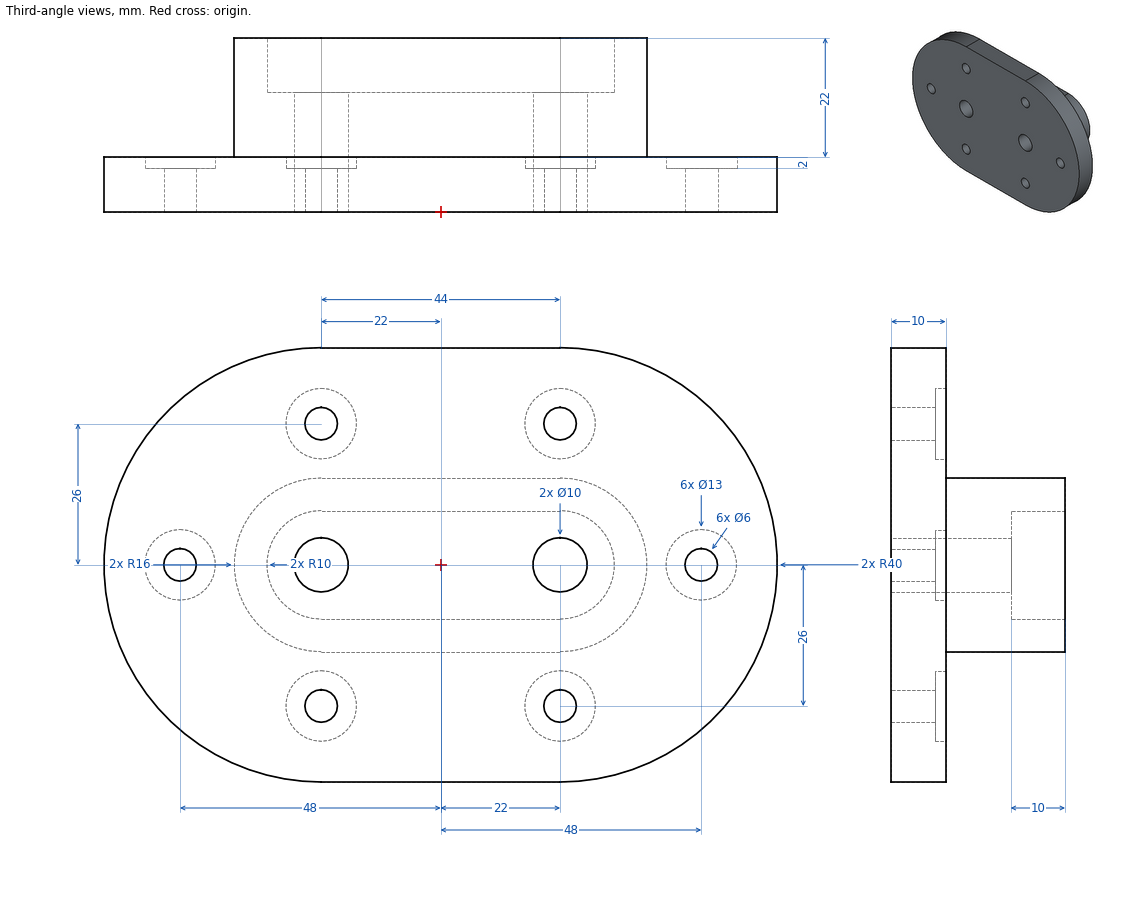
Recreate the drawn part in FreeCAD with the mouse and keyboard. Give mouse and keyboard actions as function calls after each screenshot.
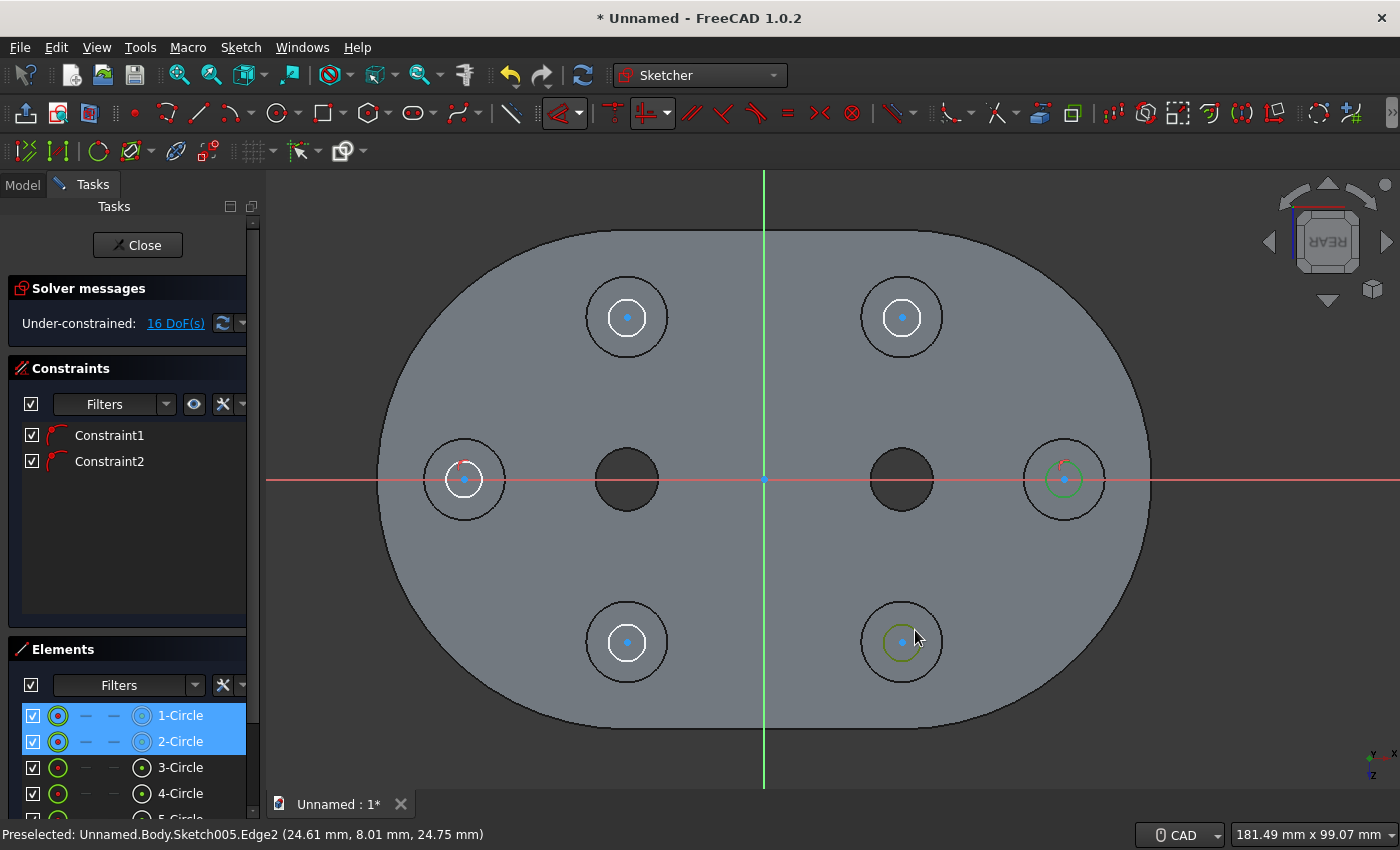
click(640, 630)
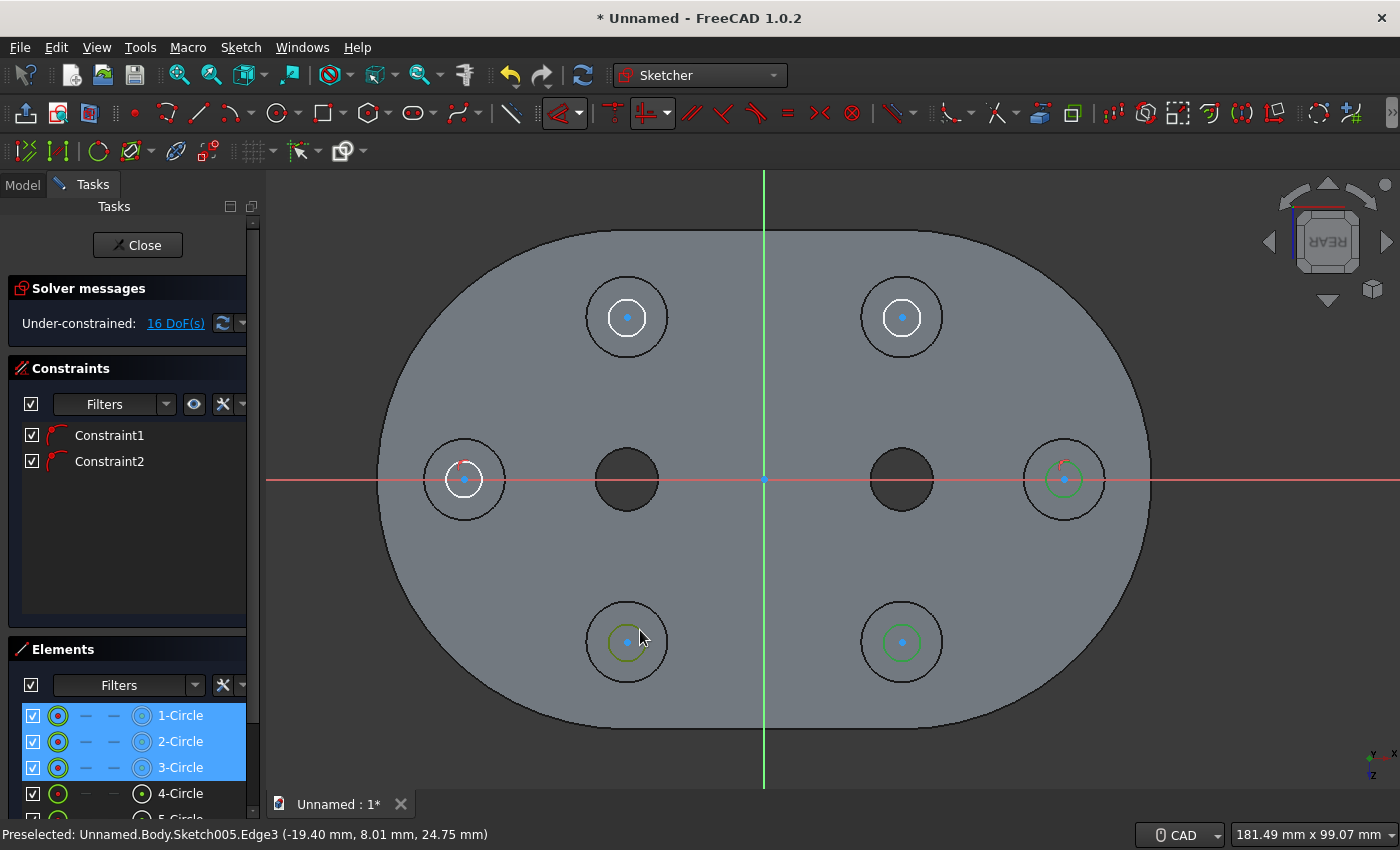
click(477, 467)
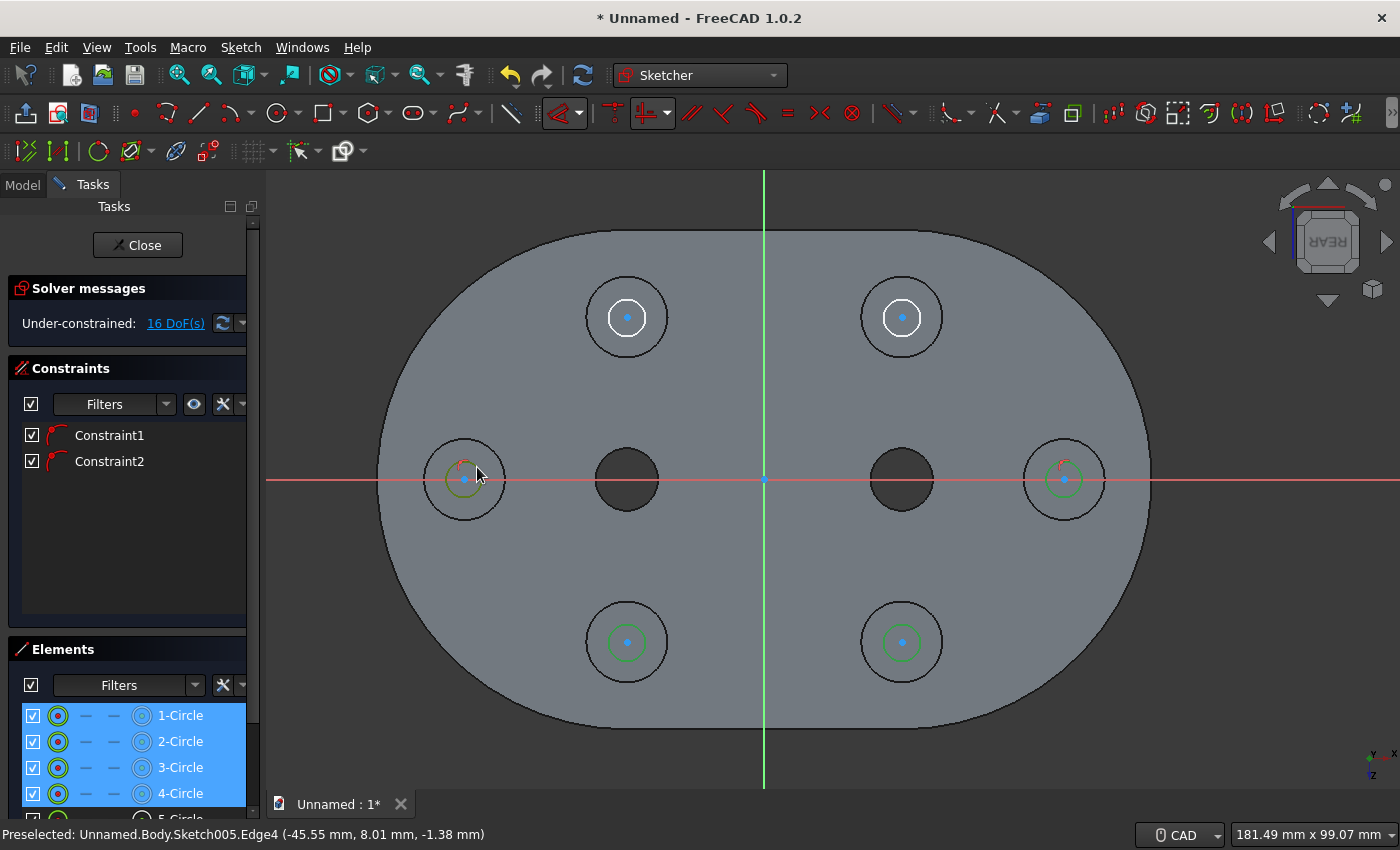
click(640, 305)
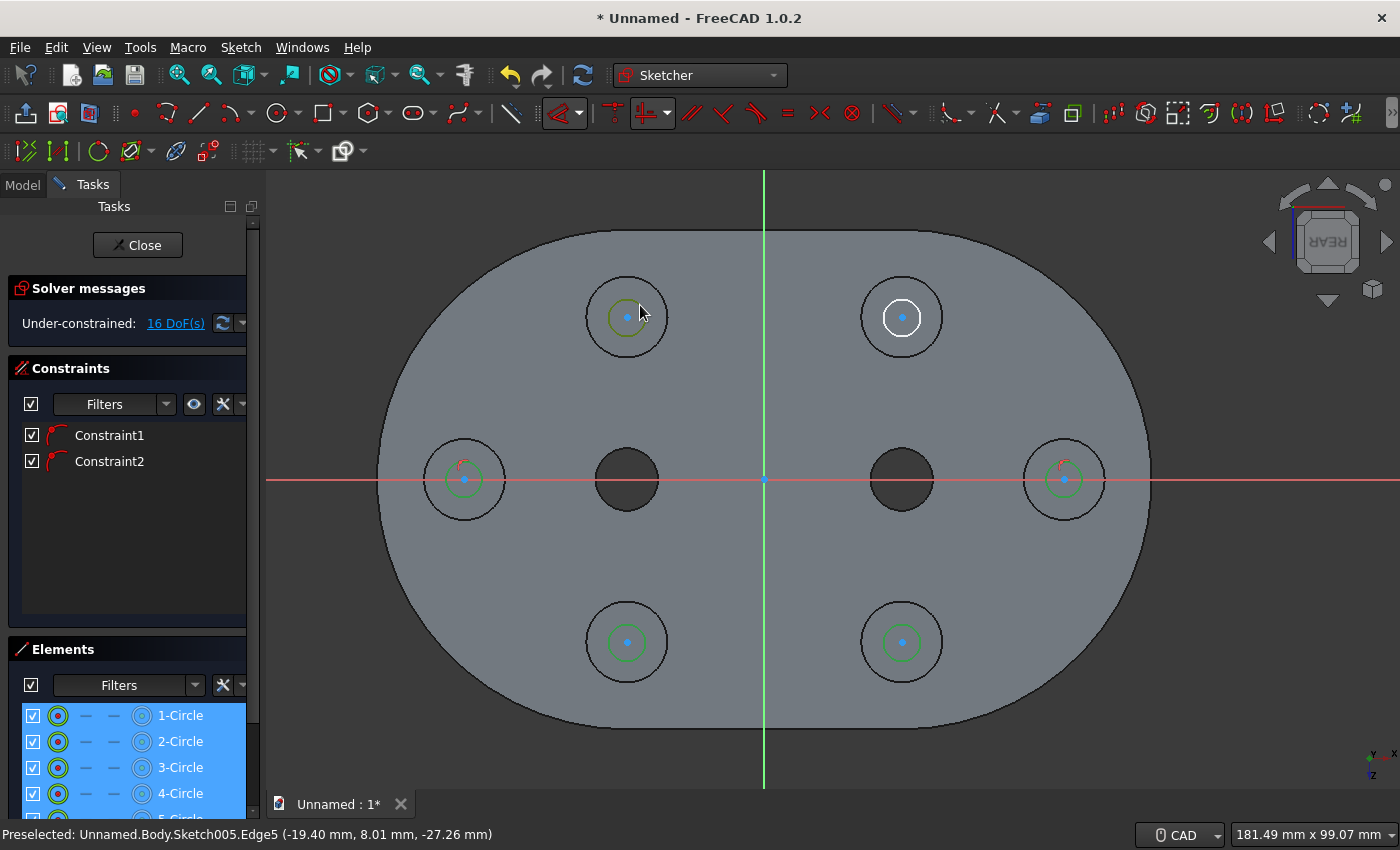
click(915, 305)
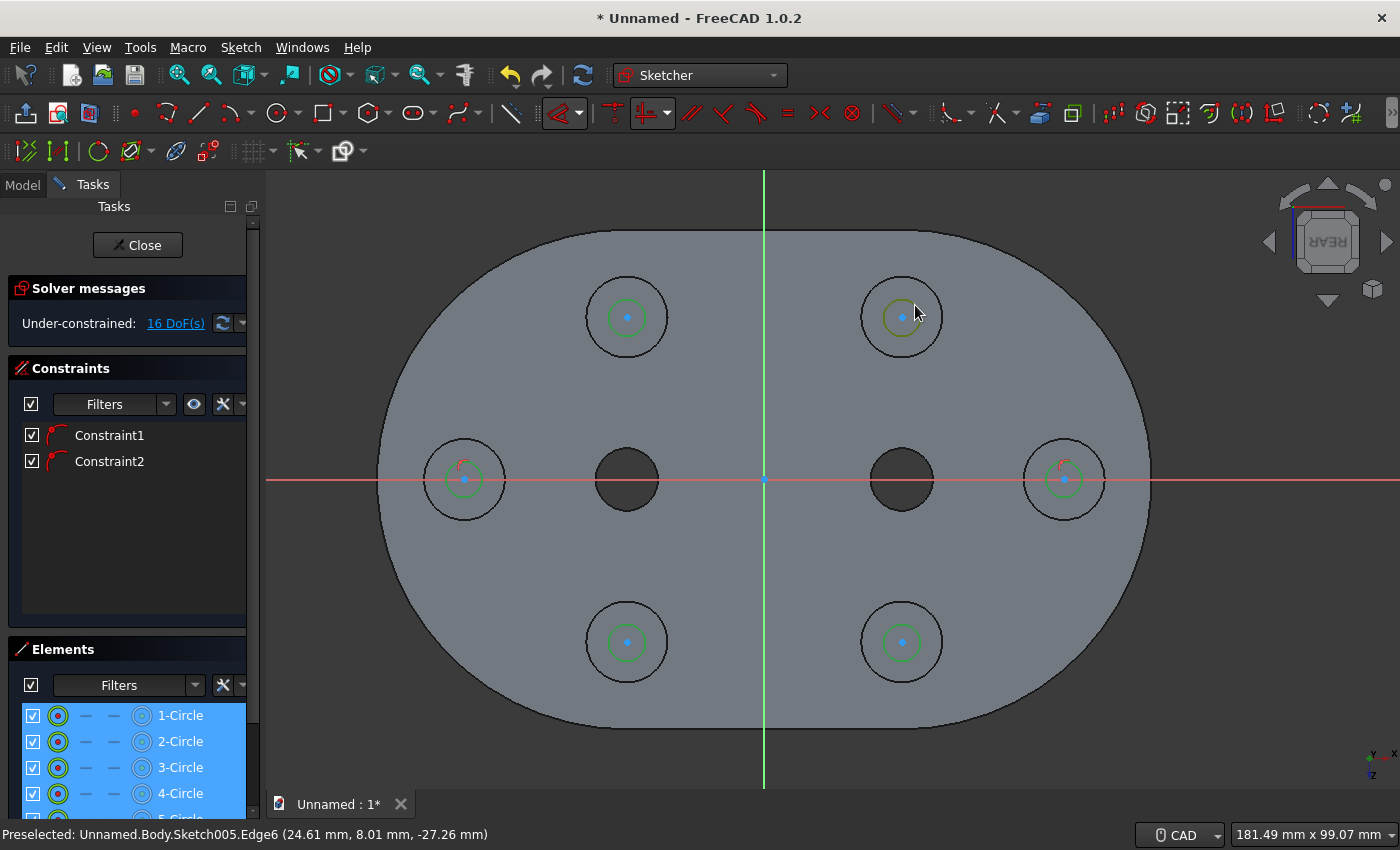
click(788, 114)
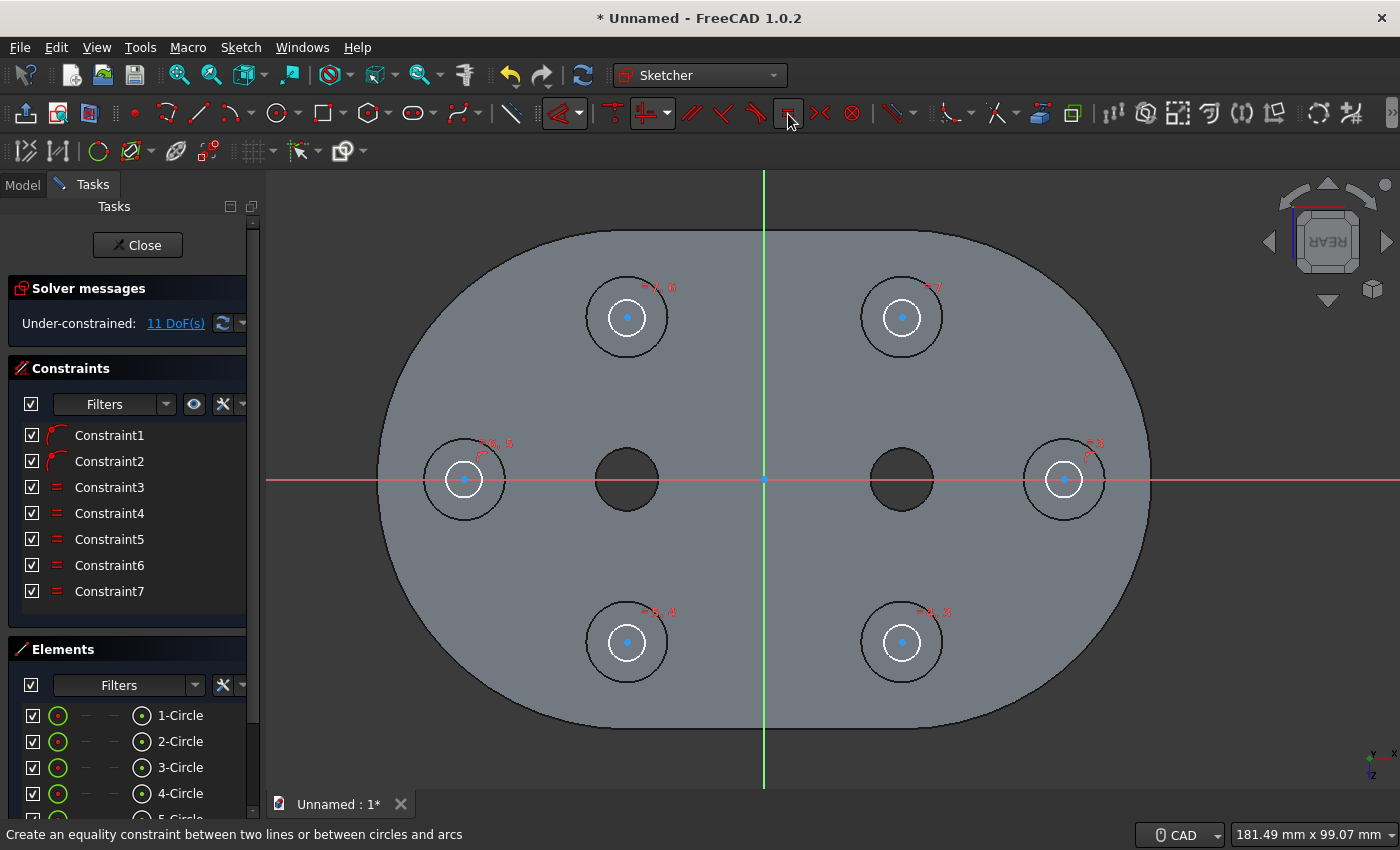
click(902, 643)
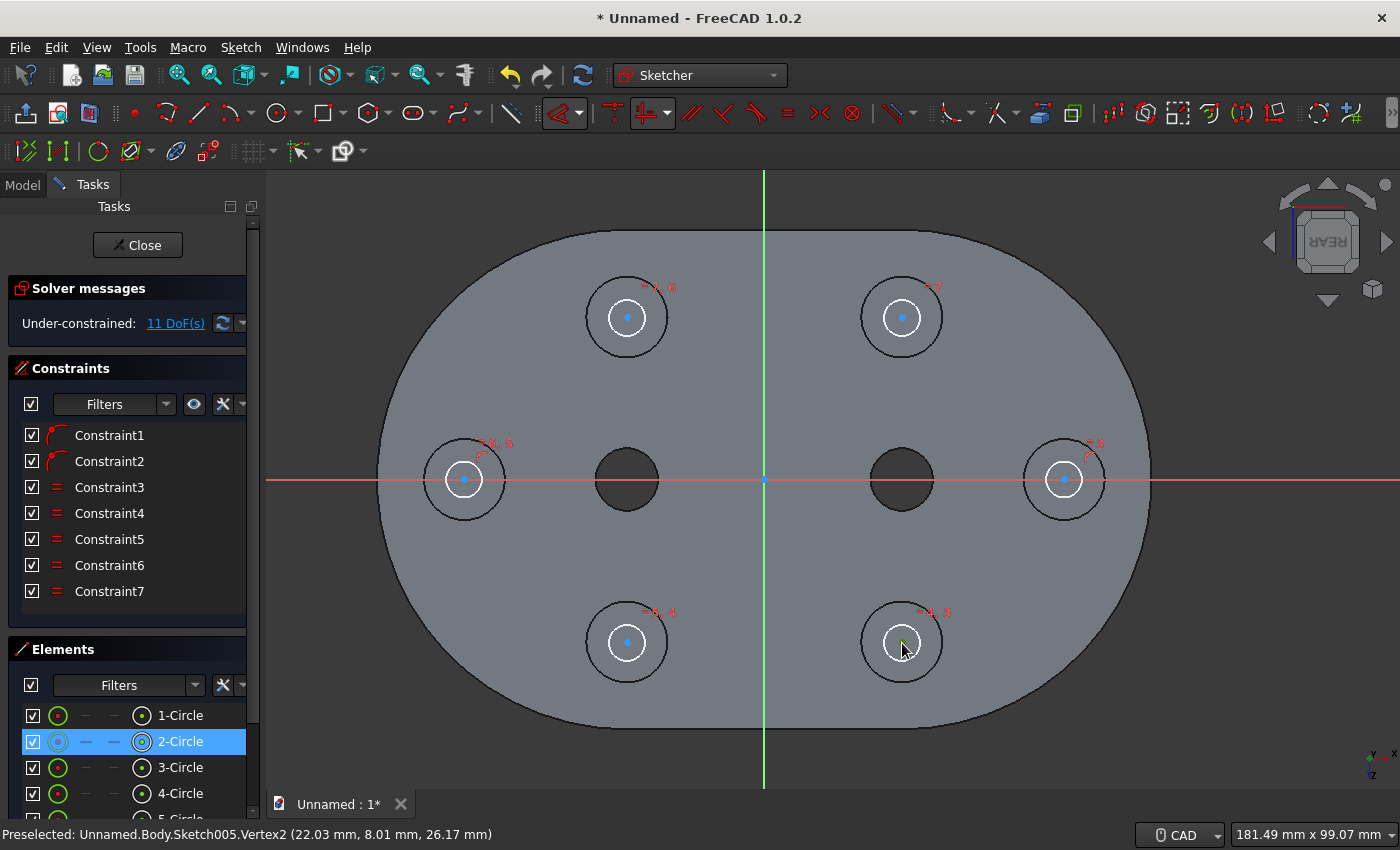
click(627, 643)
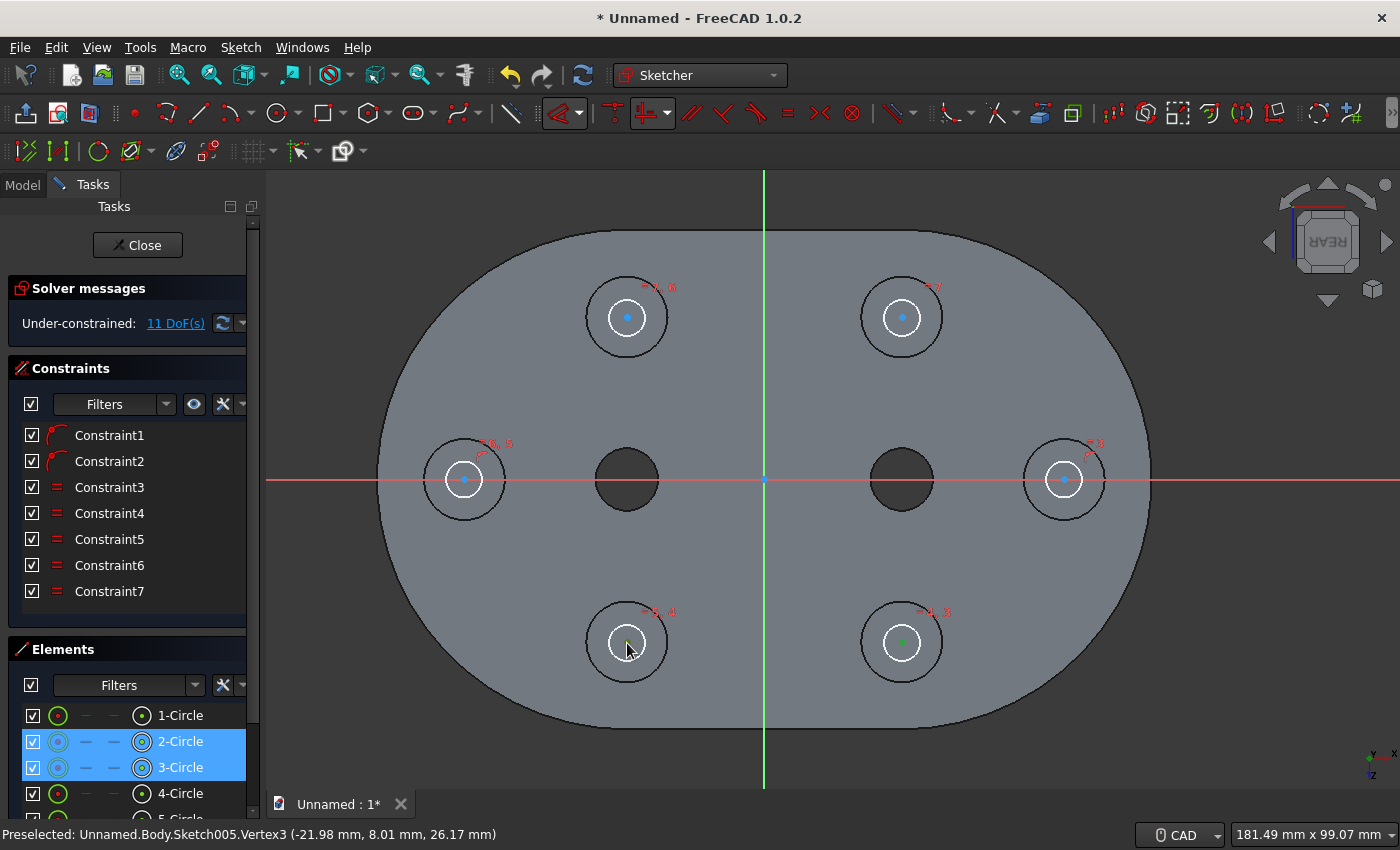
key(h)